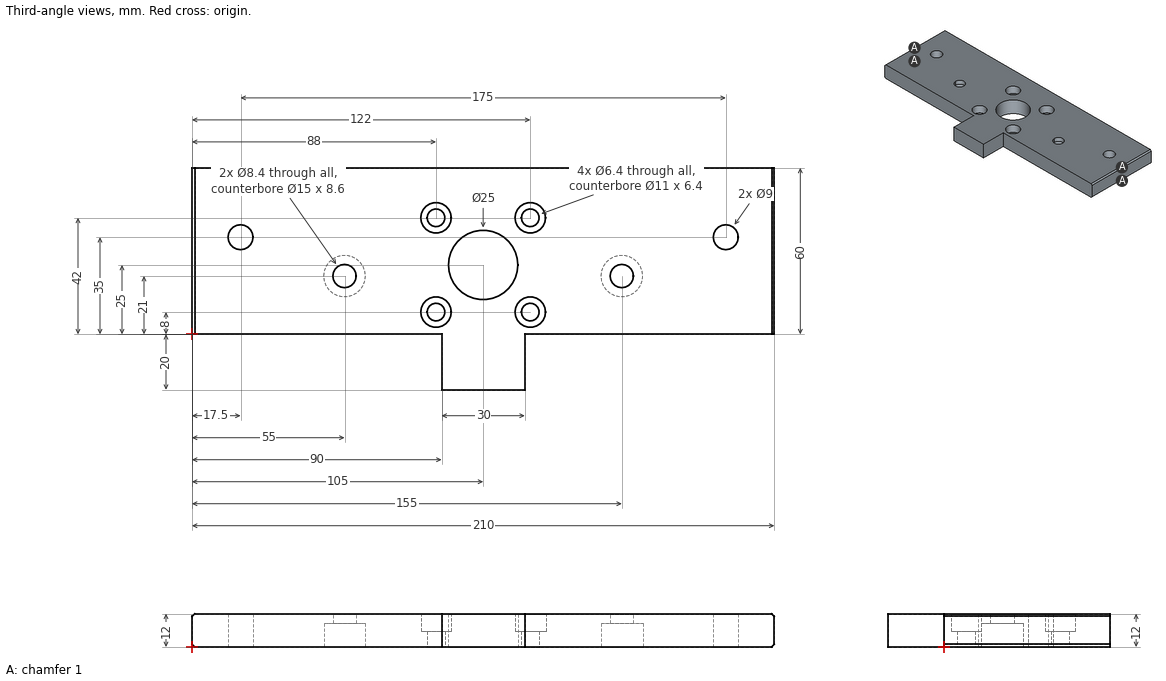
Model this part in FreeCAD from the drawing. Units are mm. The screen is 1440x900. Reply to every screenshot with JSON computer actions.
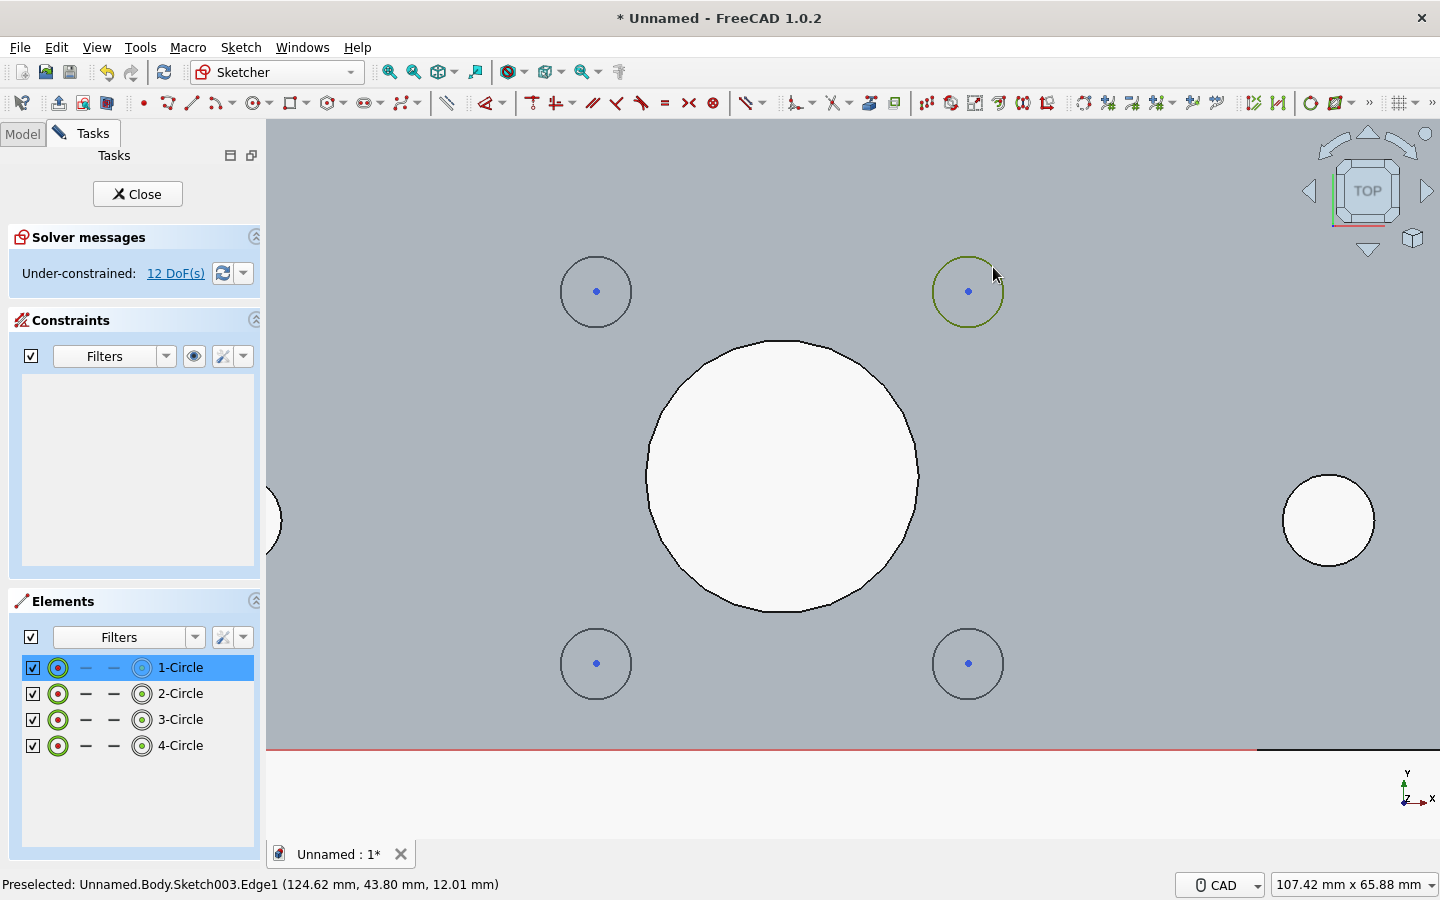
{"action": "left_click", "coordinate": [621, 267]}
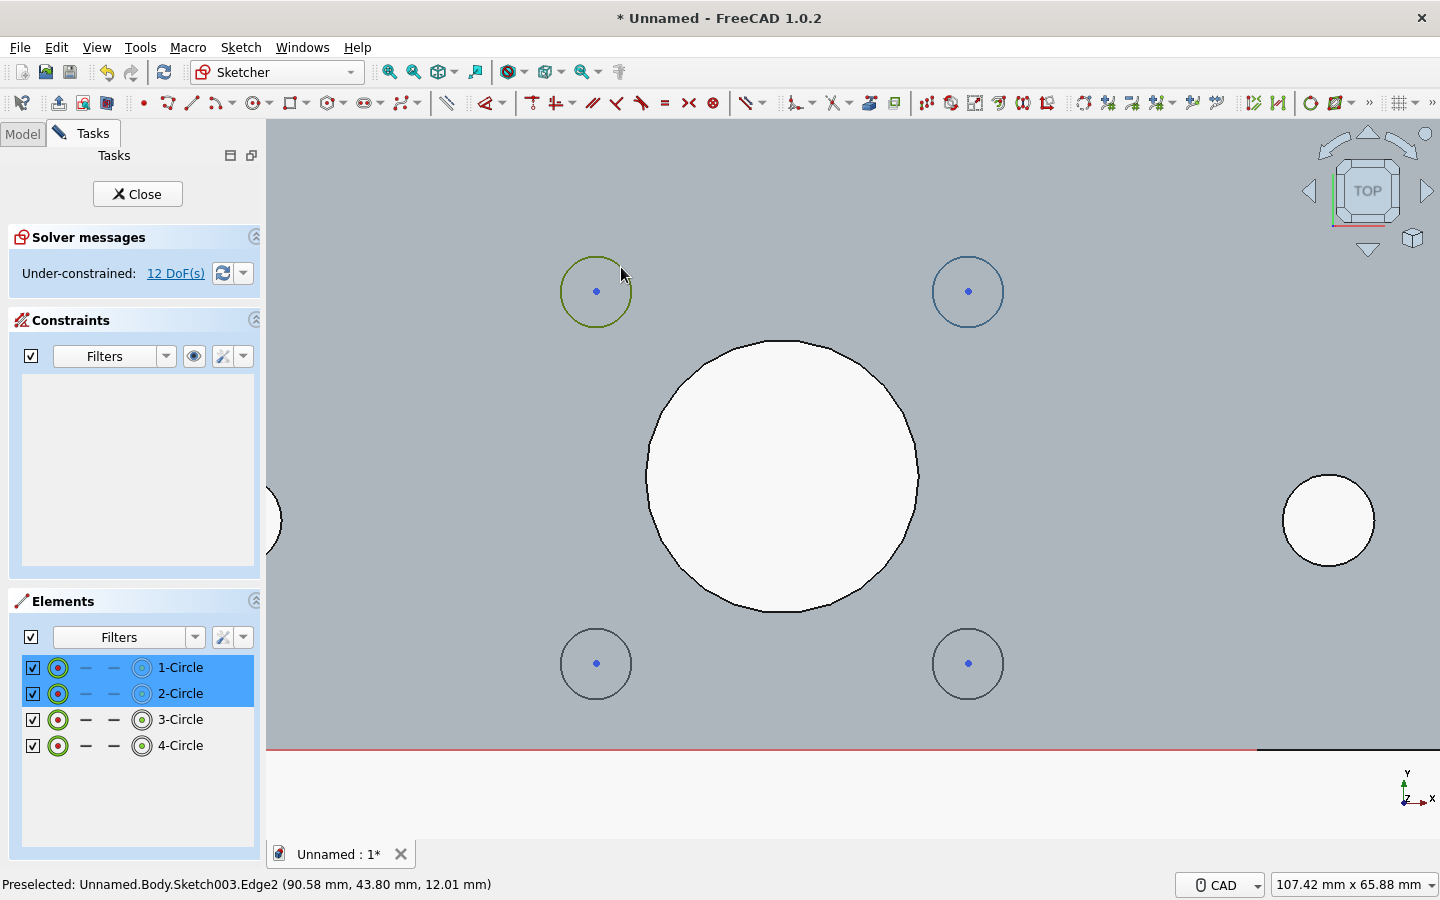
{"action": "left_click", "coordinate": [993, 639]}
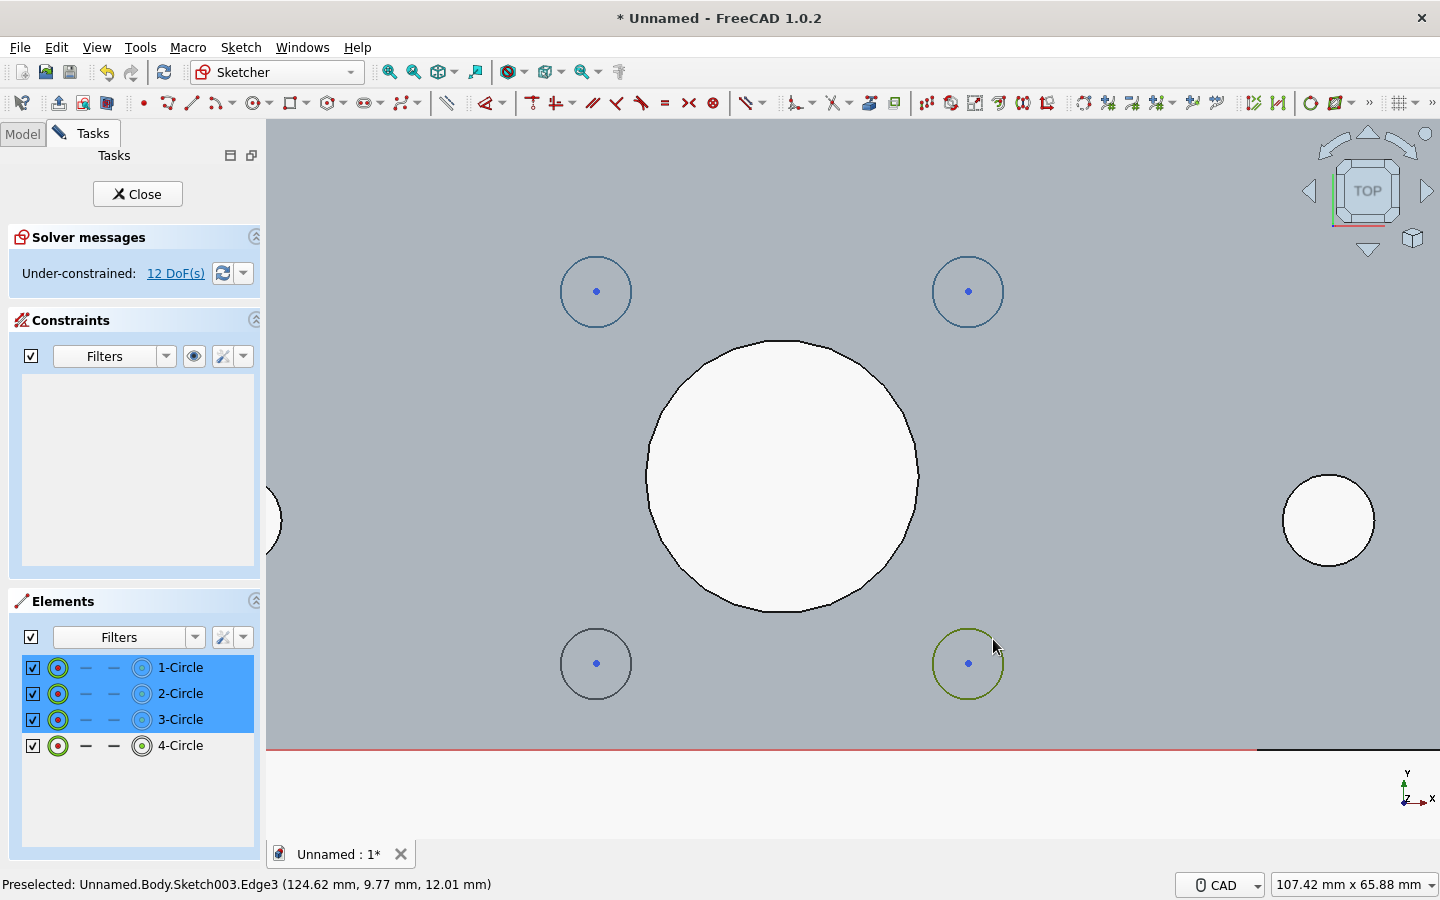
{"action": "left_click", "coordinate": [621, 639]}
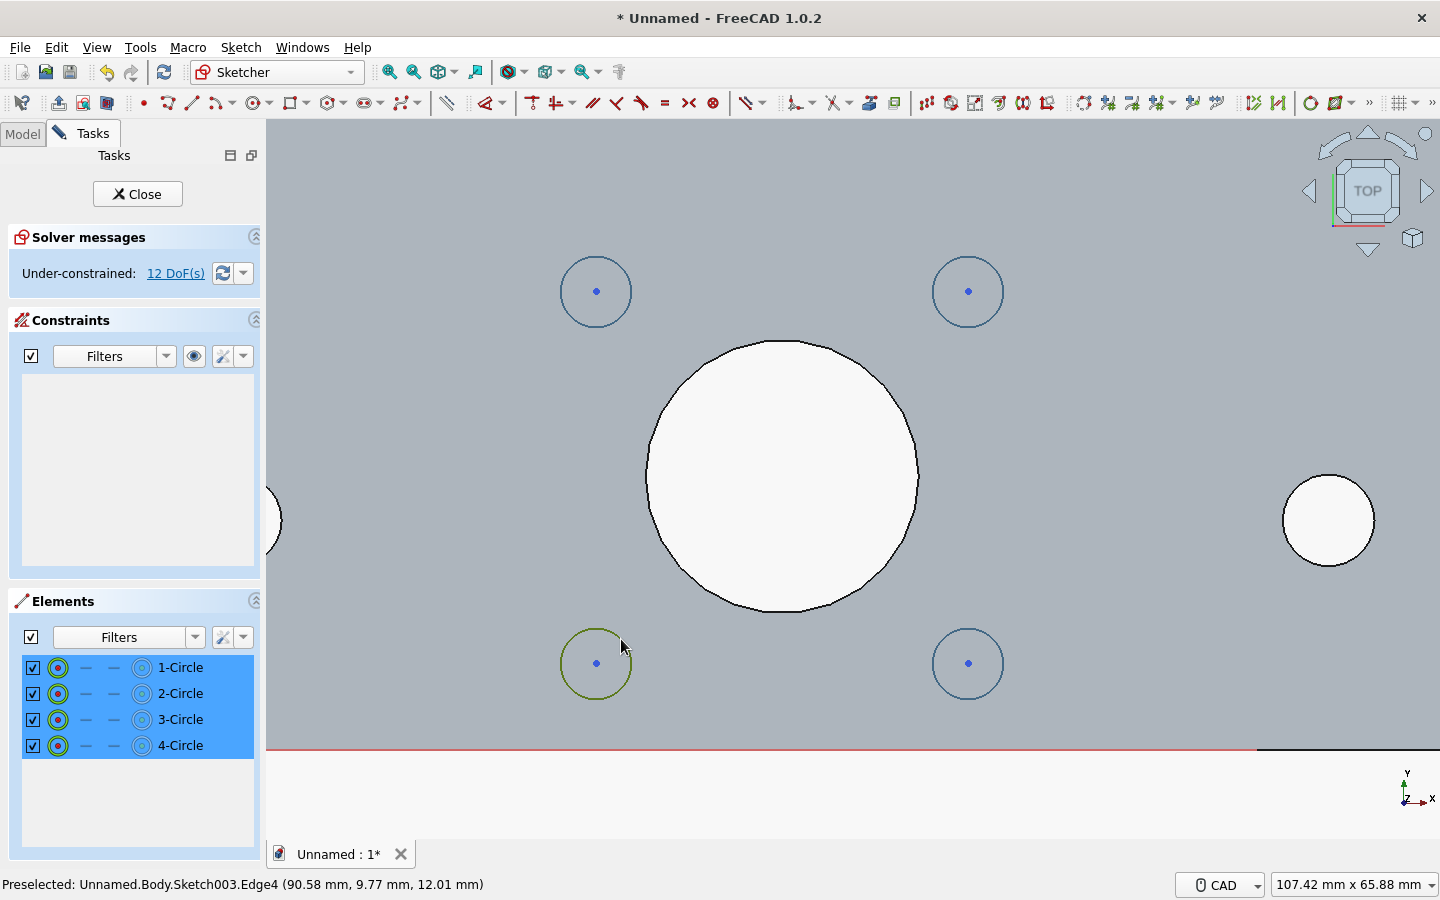
{"action": "key", "text": "e"}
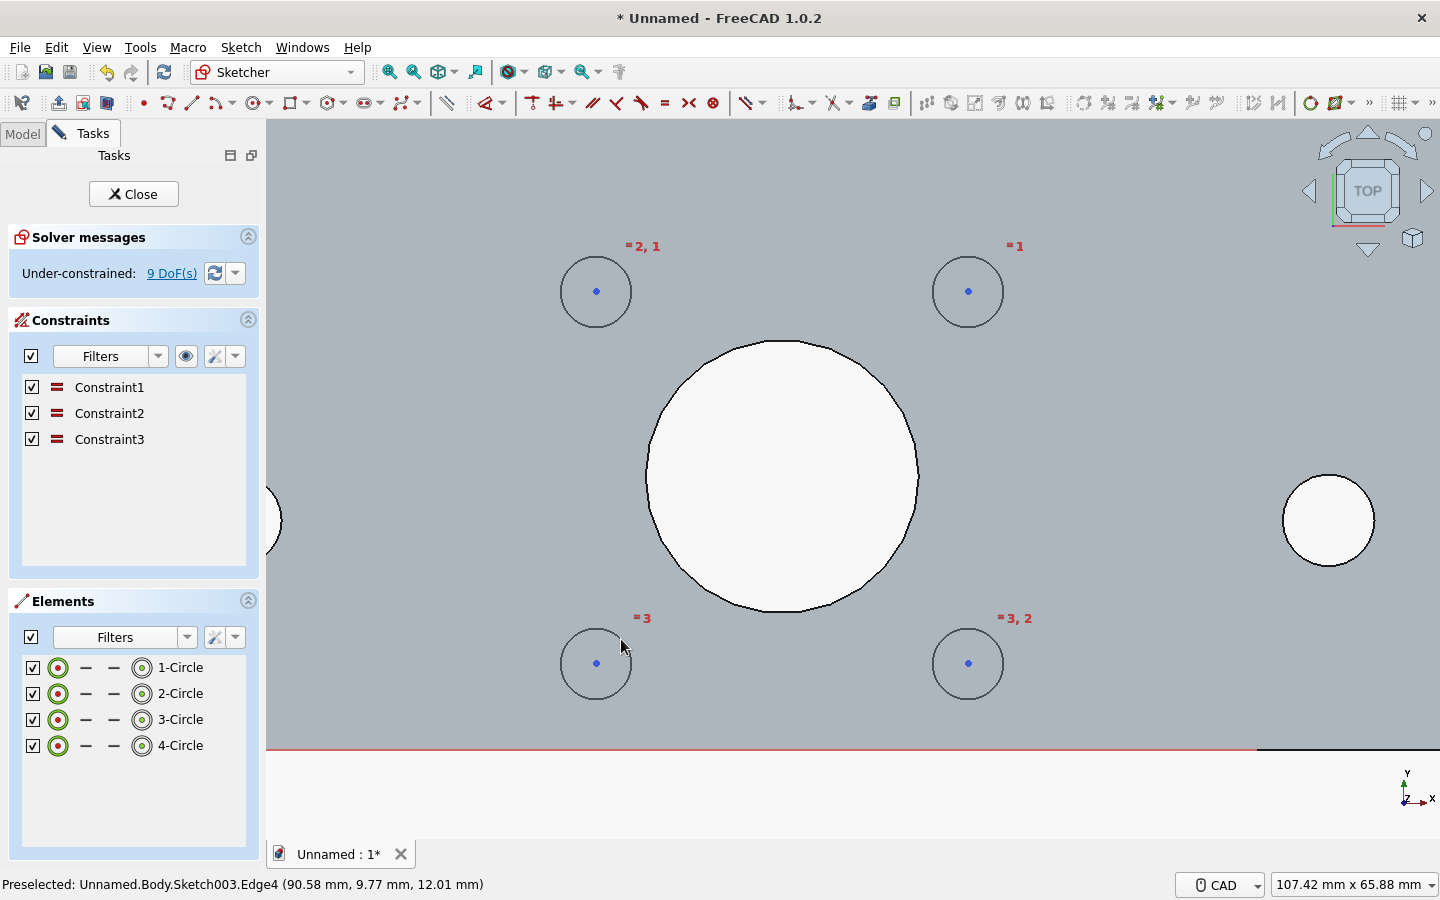
{"action": "left_click", "coordinate": [968, 292]}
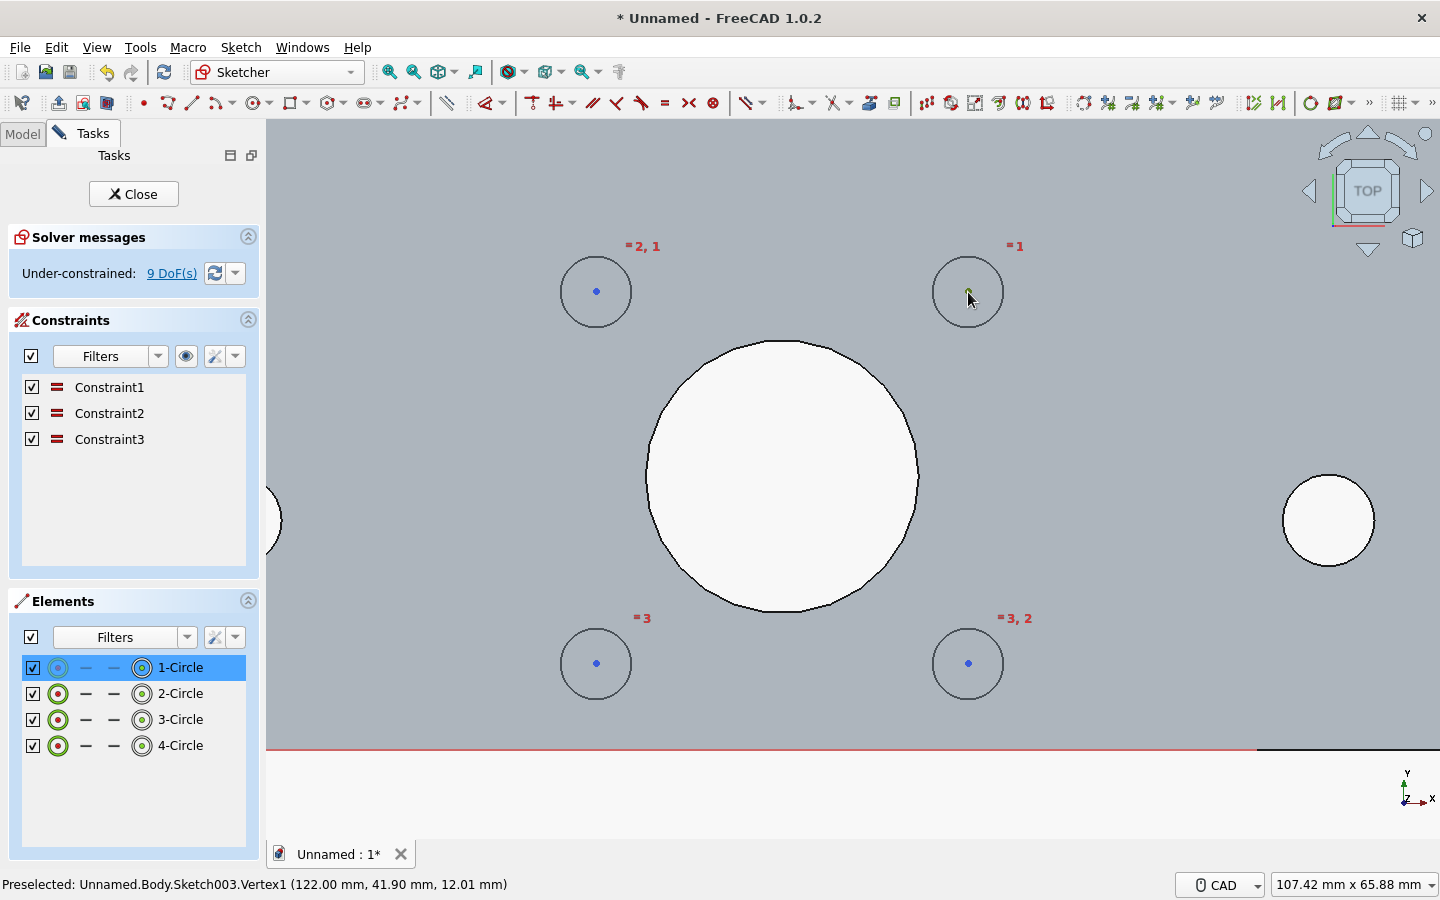
{"action": "left_click", "coordinate": [596, 292]}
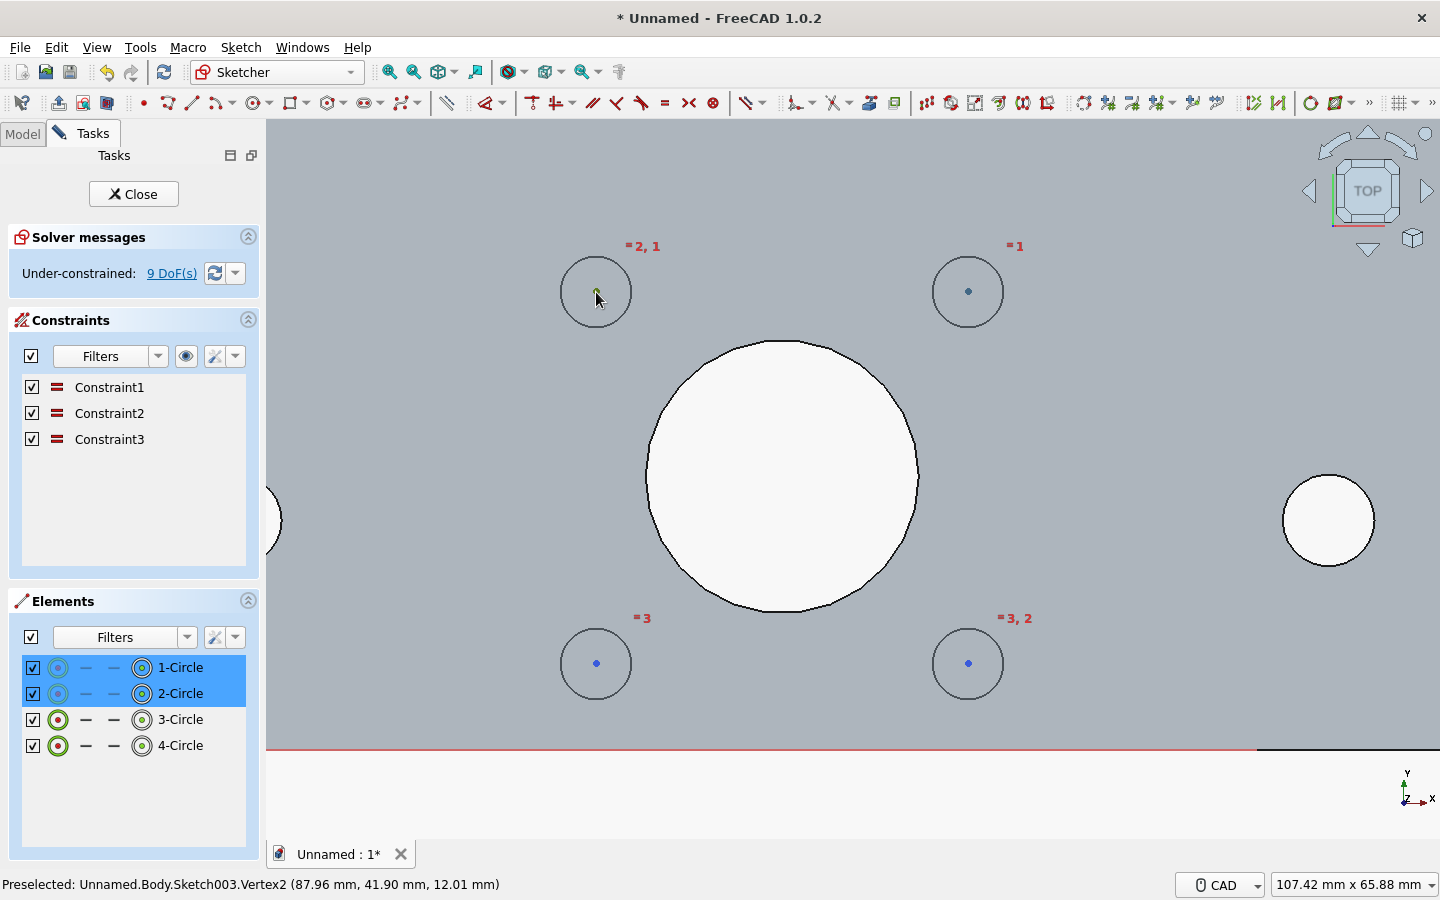
{"action": "key", "text": "h"}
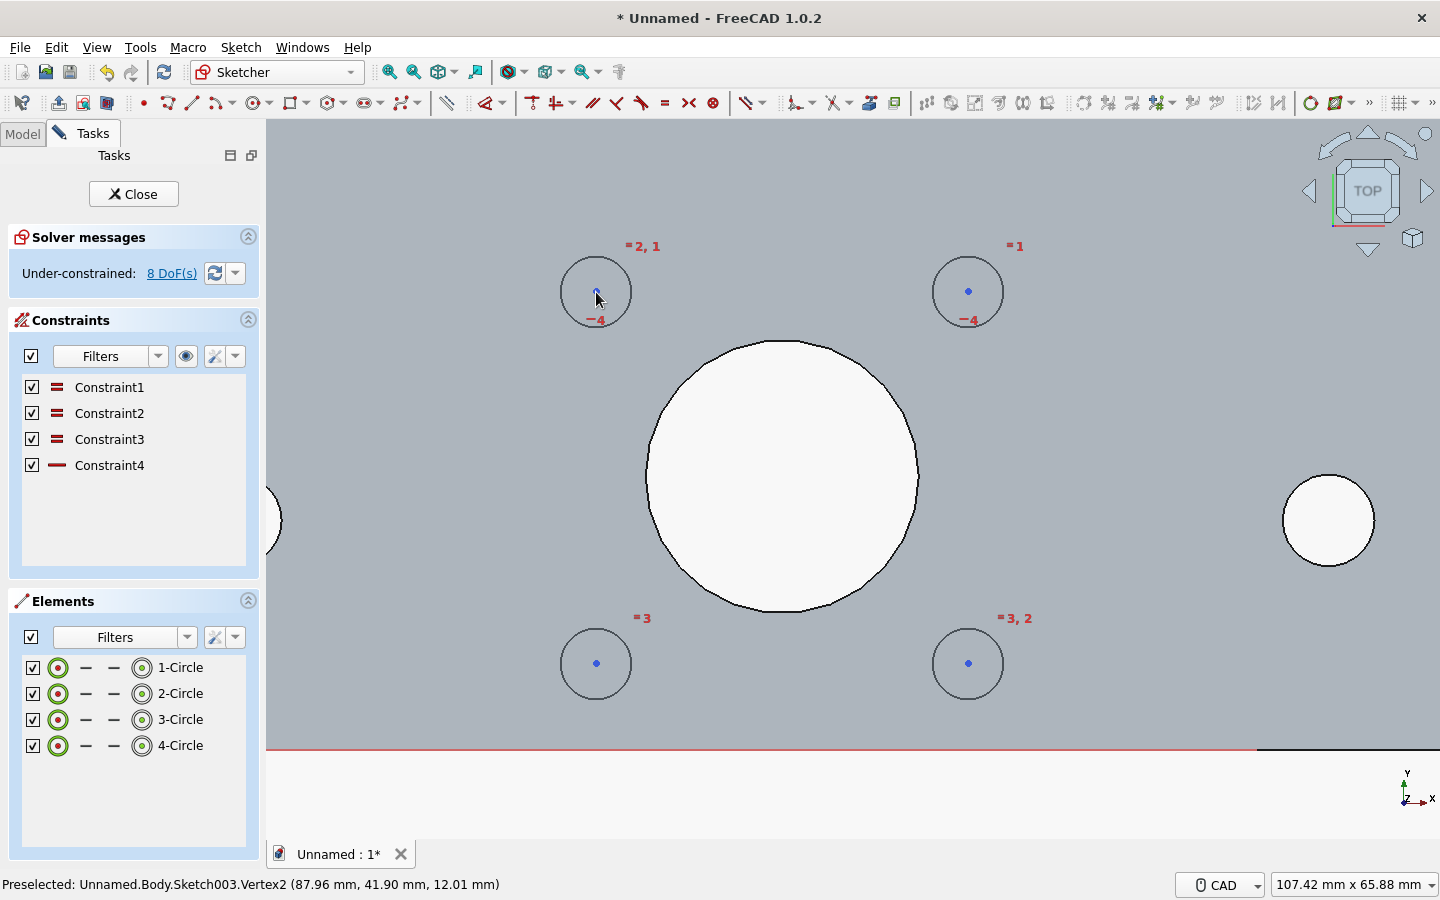
{"action": "left_click", "coordinate": [968, 292]}